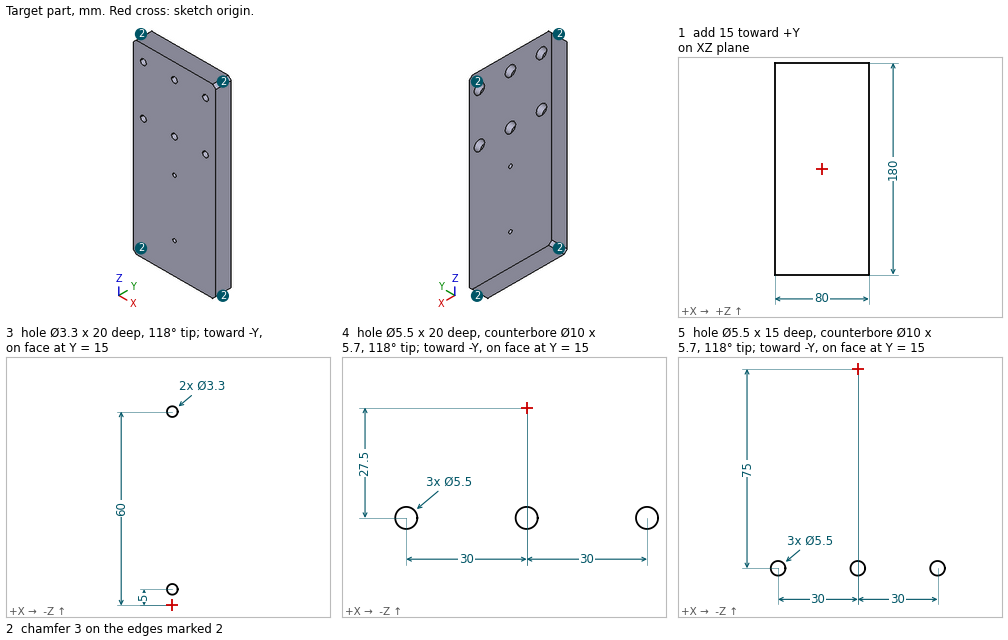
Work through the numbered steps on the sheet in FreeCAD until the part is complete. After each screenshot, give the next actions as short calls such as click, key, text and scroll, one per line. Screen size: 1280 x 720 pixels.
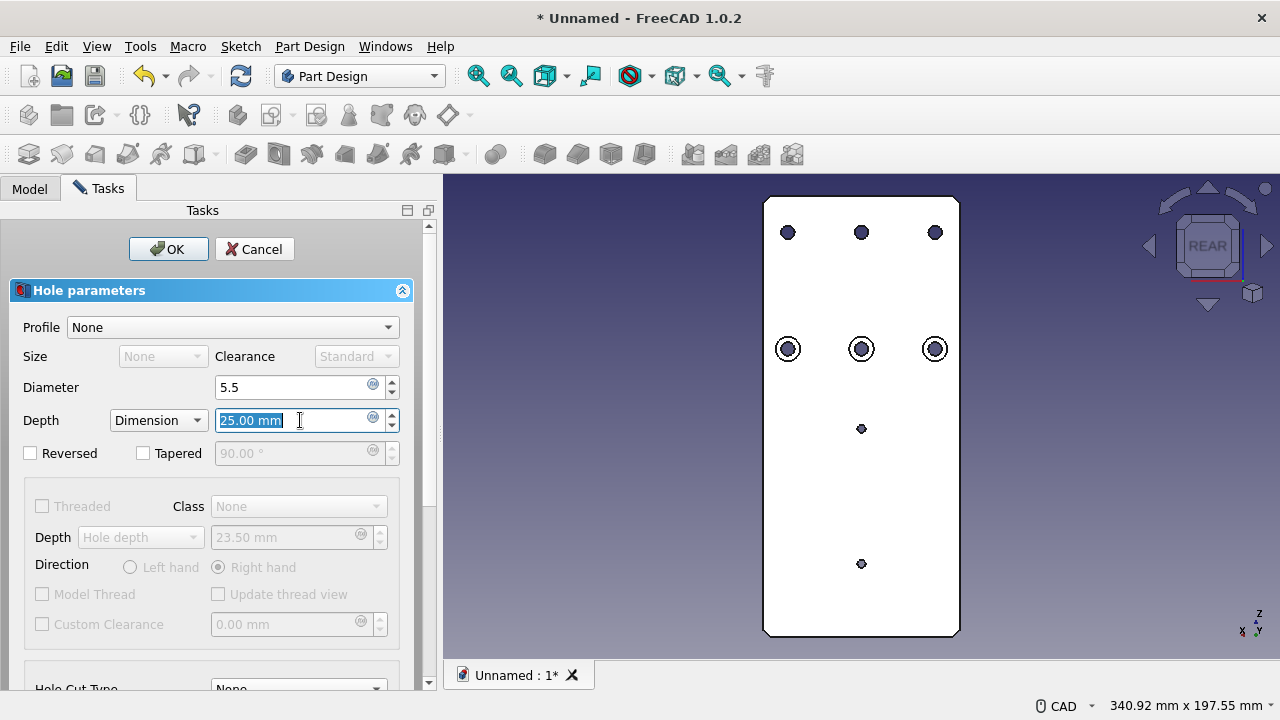
text(15)
key(Tab)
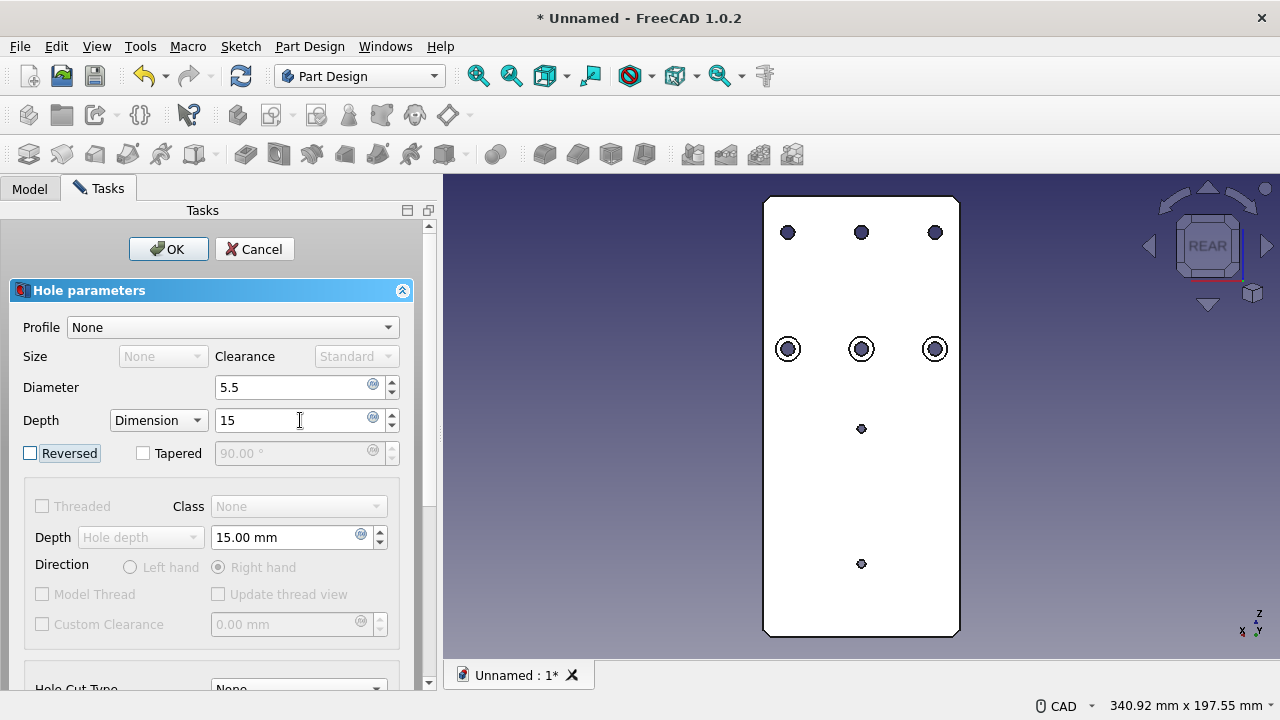
scroll(429, 455, down, 2)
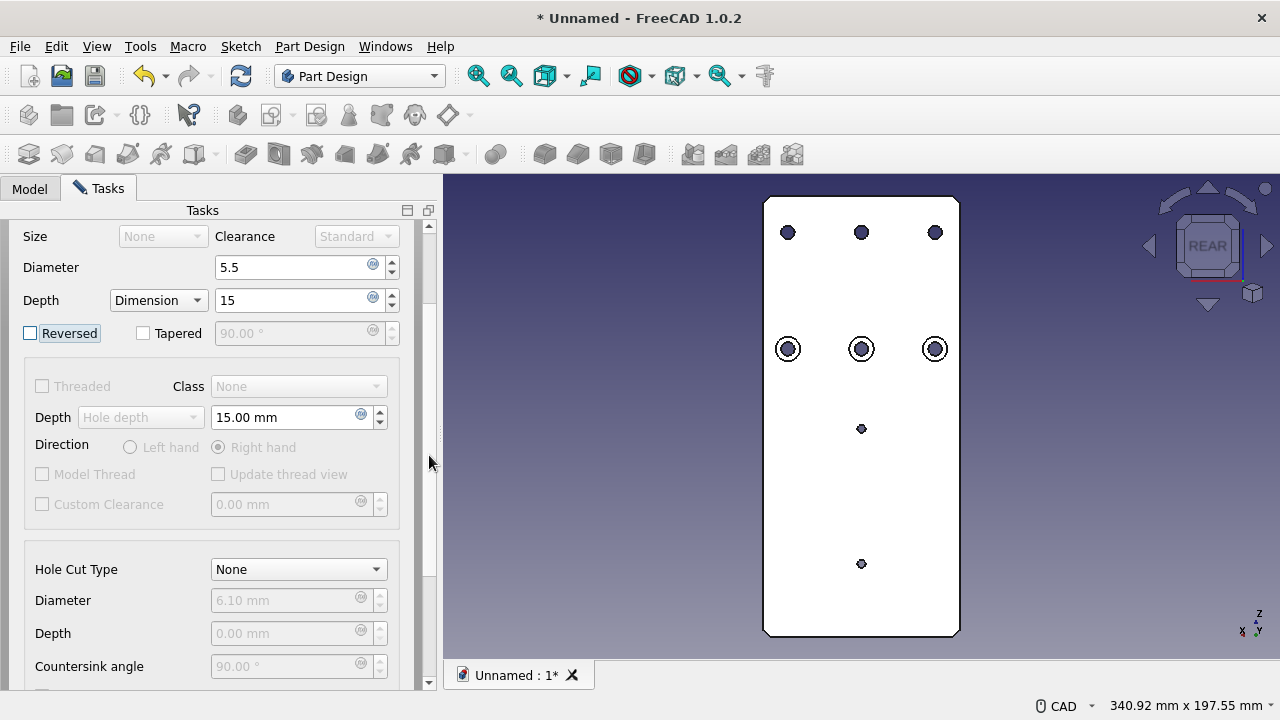
click(300, 570)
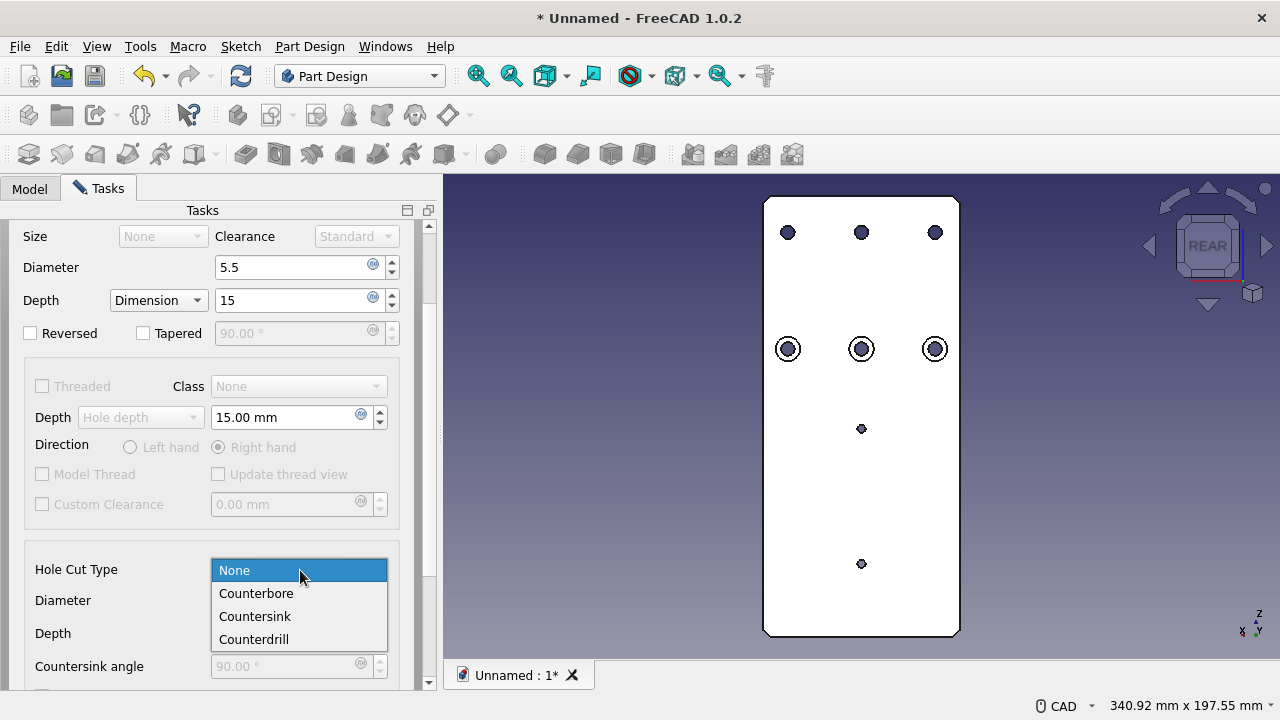
click(298, 594)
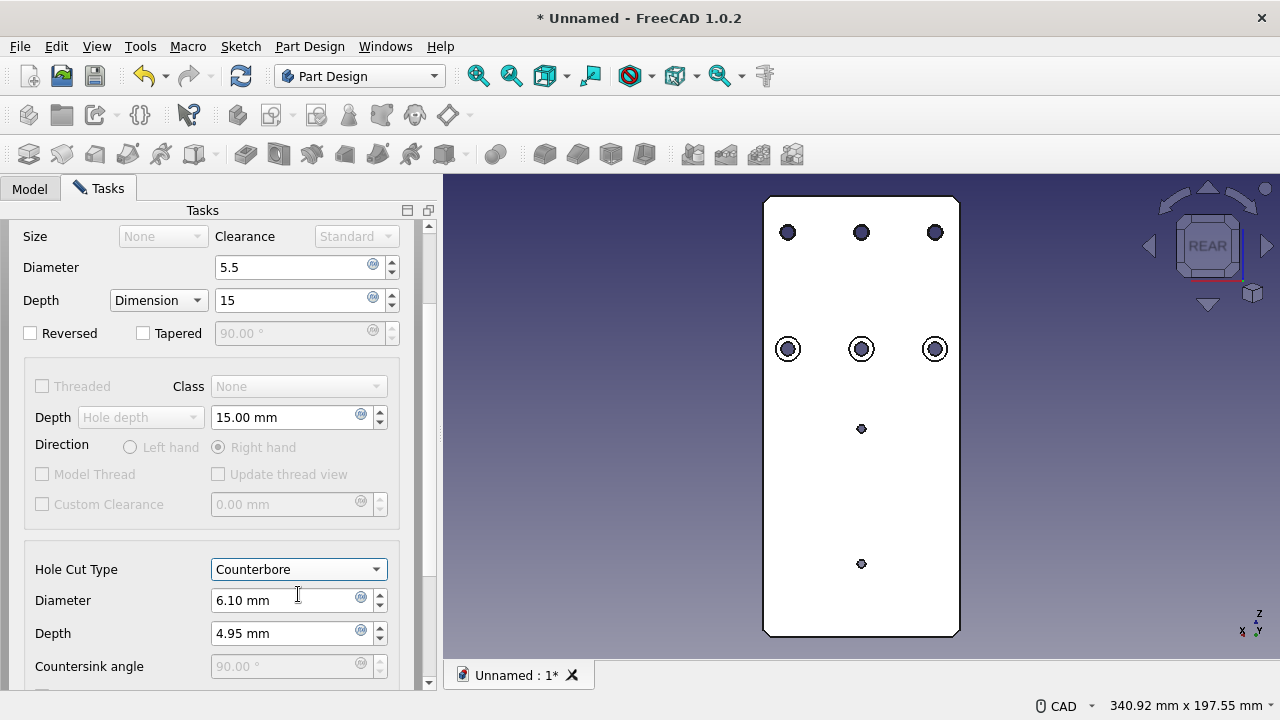
triple_click(292, 600)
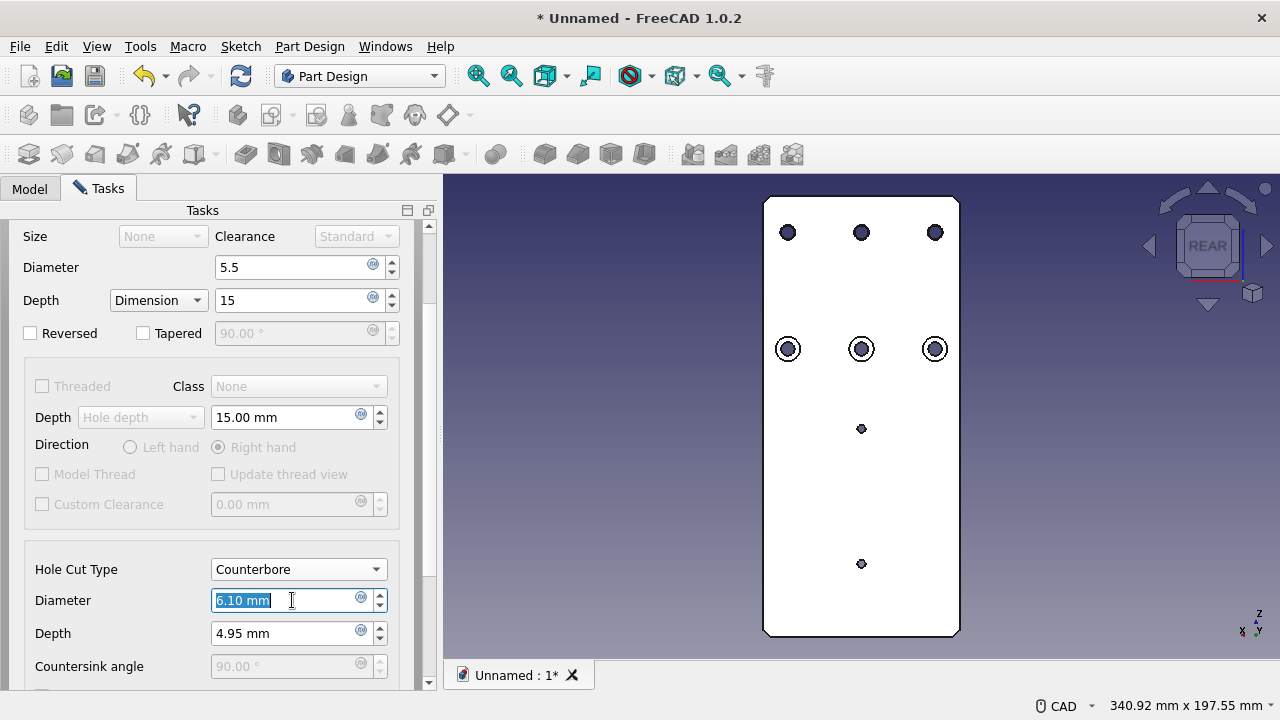
text(10)
key(Tab)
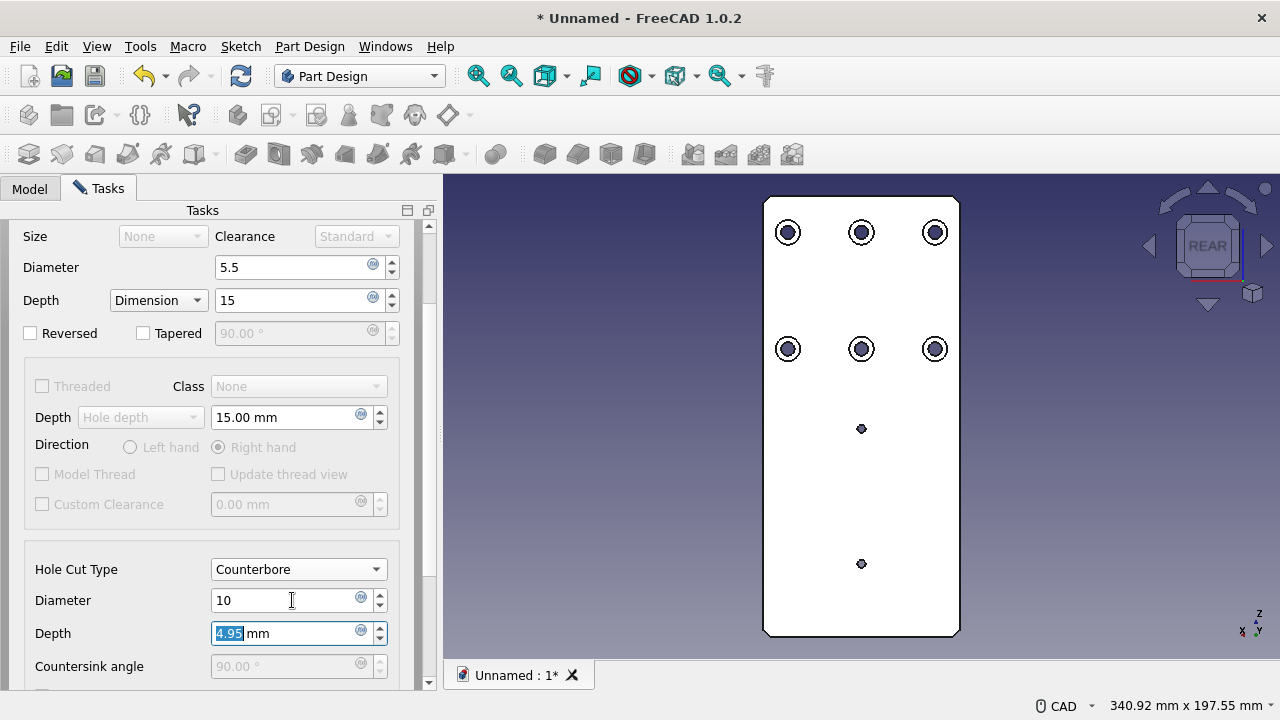
text(5.7)
key(Tab)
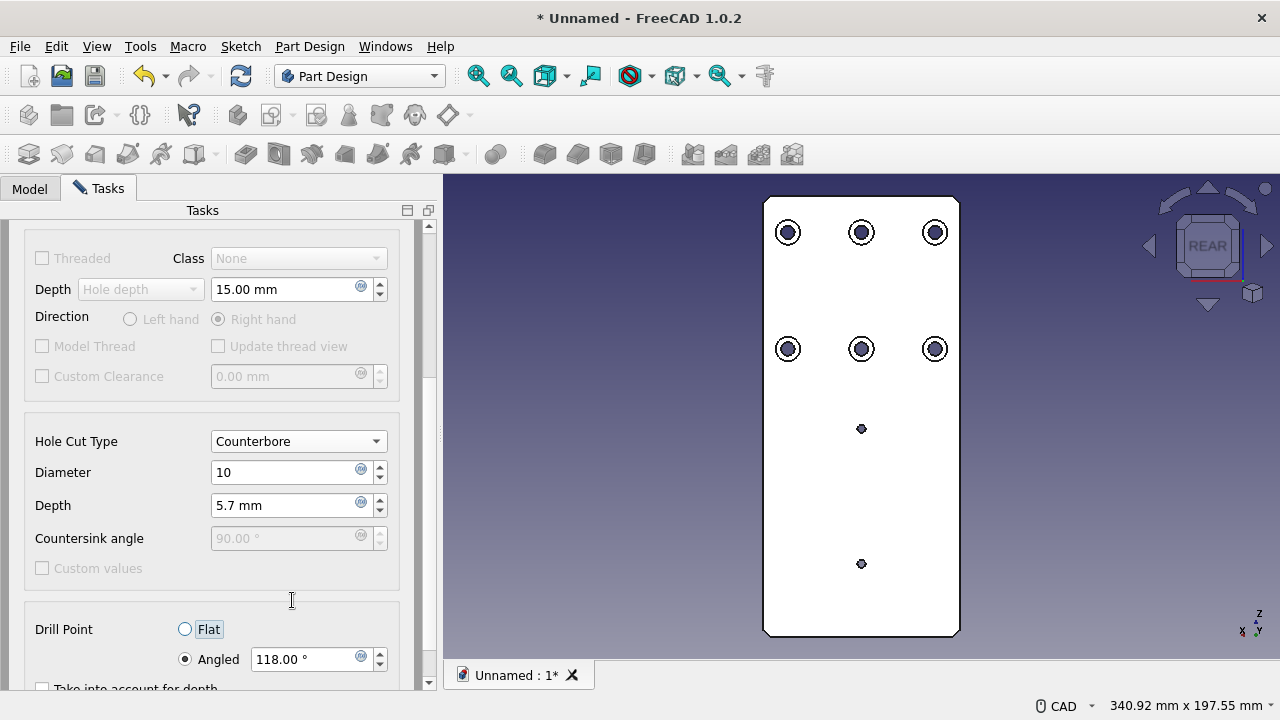
scroll(429, 455, up, 5)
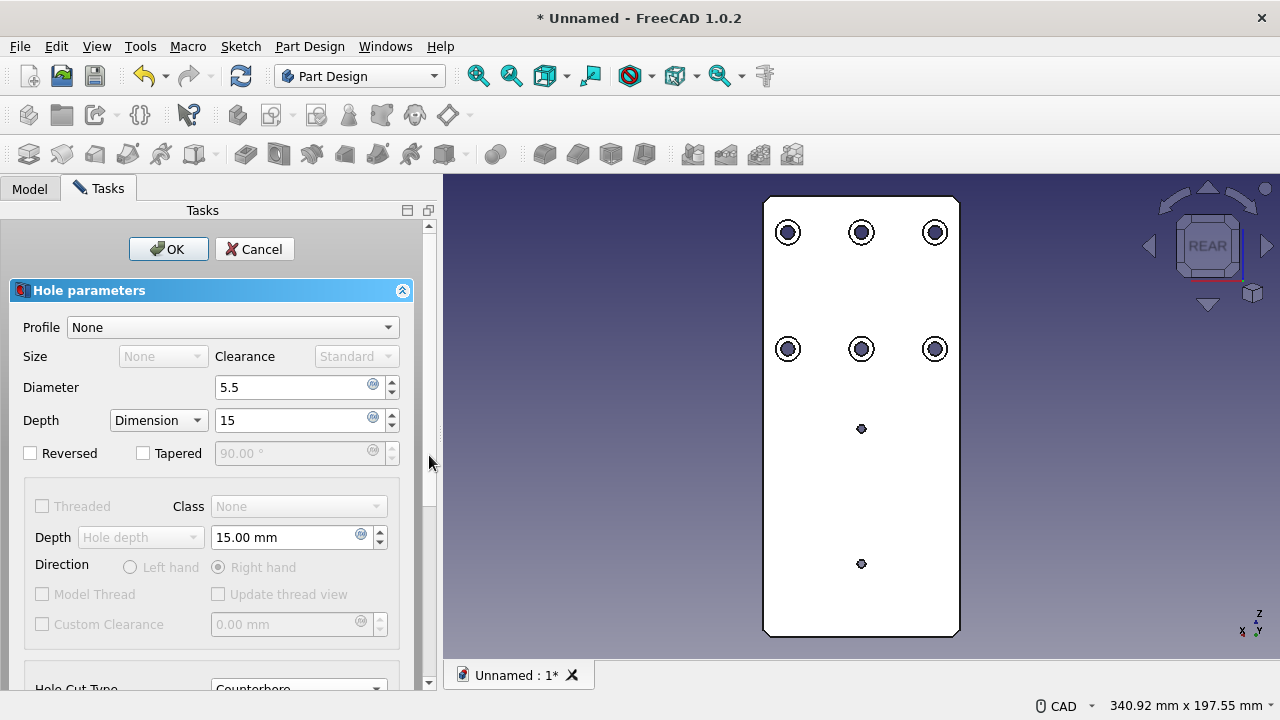
click(169, 249)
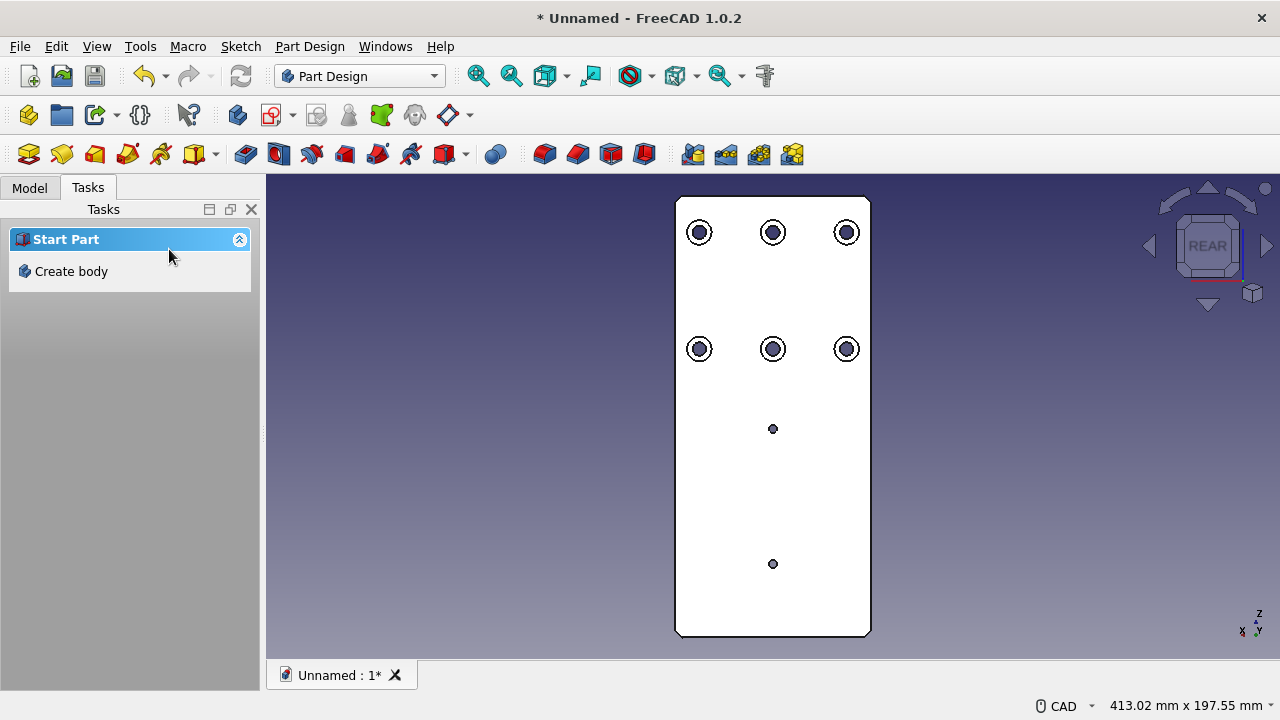
key(0)